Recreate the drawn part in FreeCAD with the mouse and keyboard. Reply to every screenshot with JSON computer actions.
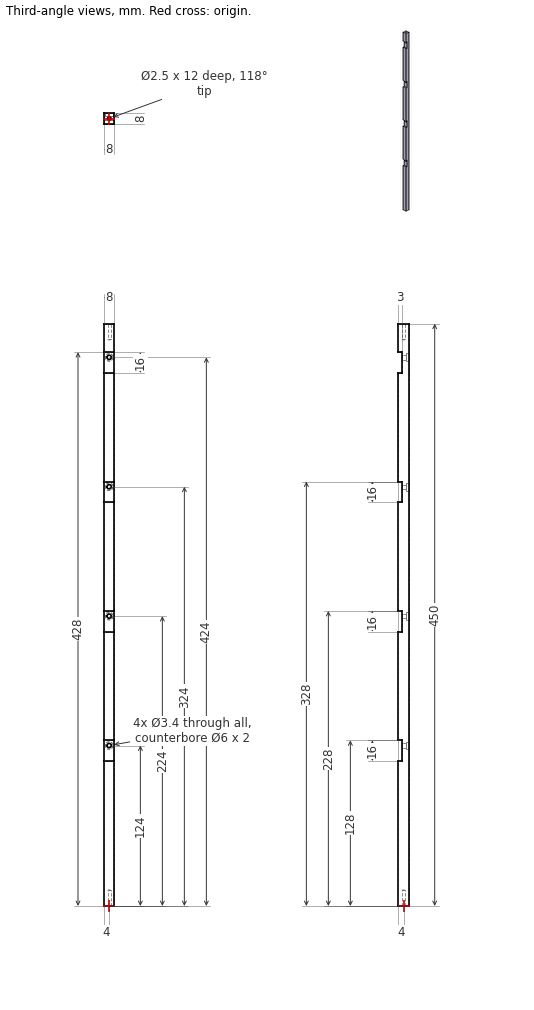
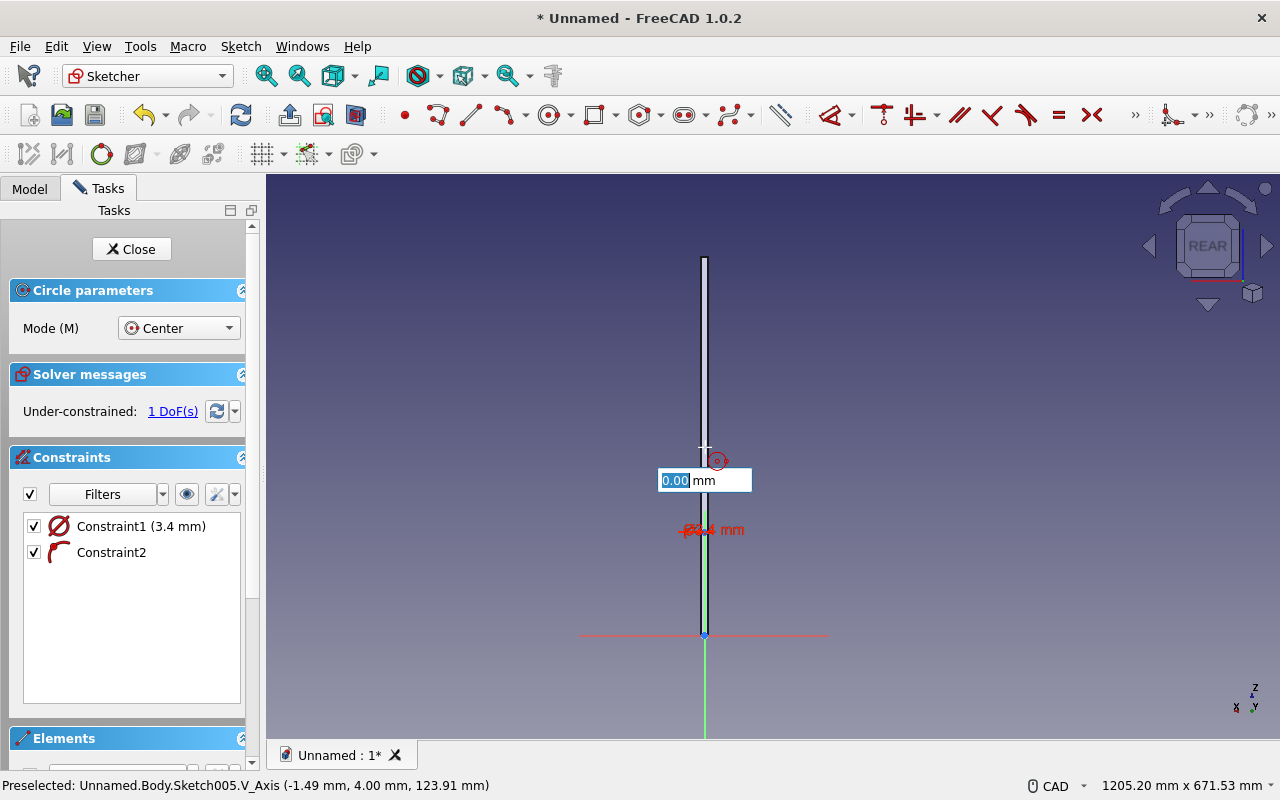
{"action": "scroll", "coordinate": [706, 447], "scroll_direction": "up", "scroll_amount": 13}
{"action": "mouse_move", "coordinate": [699, 436]}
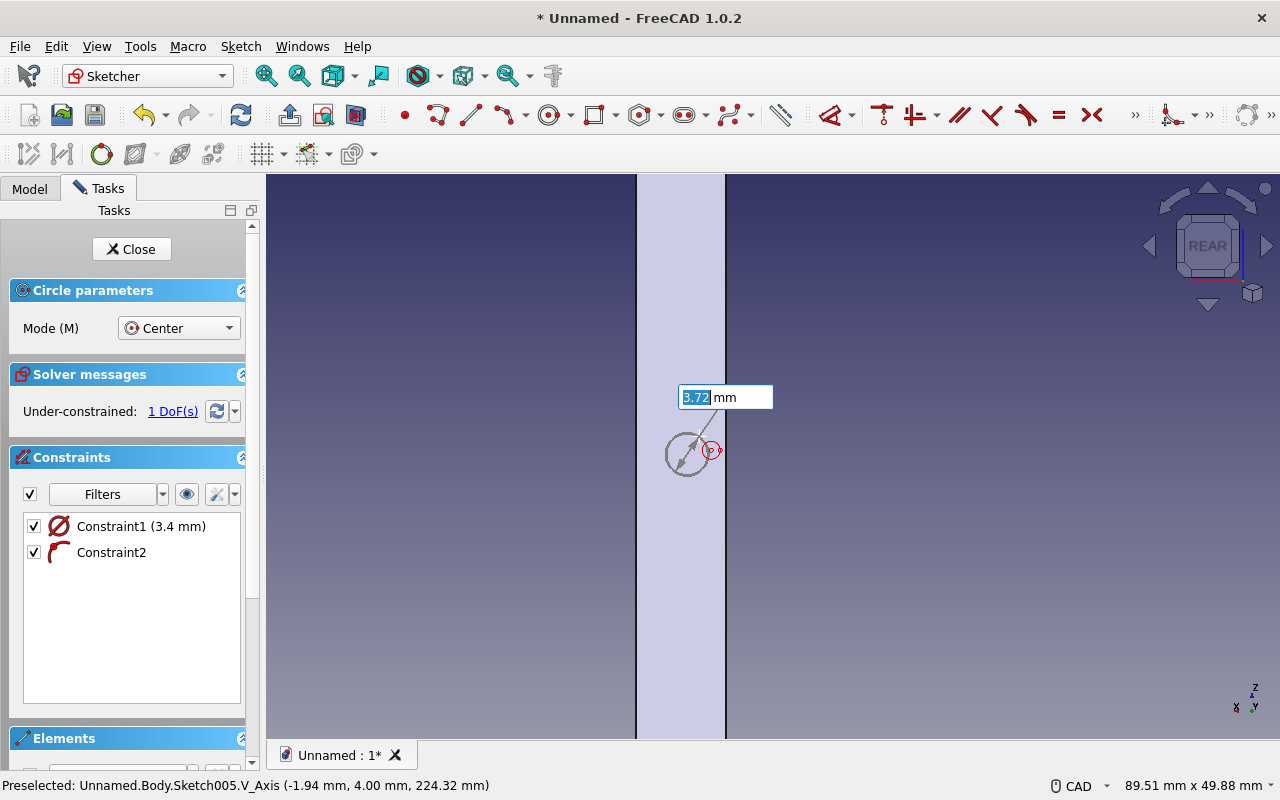
{"action": "type", "text": "3.4"}
{"action": "key", "text": "Return"}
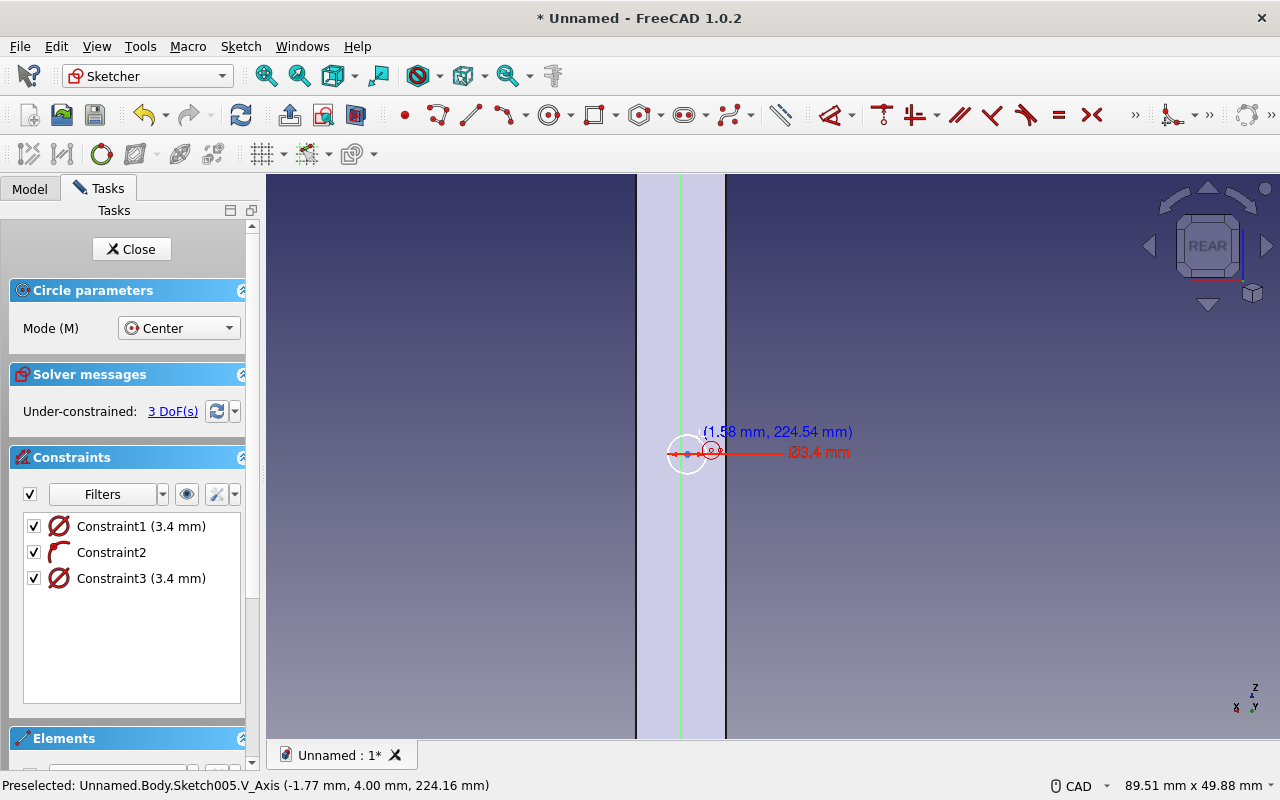
{"action": "scroll", "coordinate": [706, 447], "scroll_direction": "down", "scroll_amount": 13}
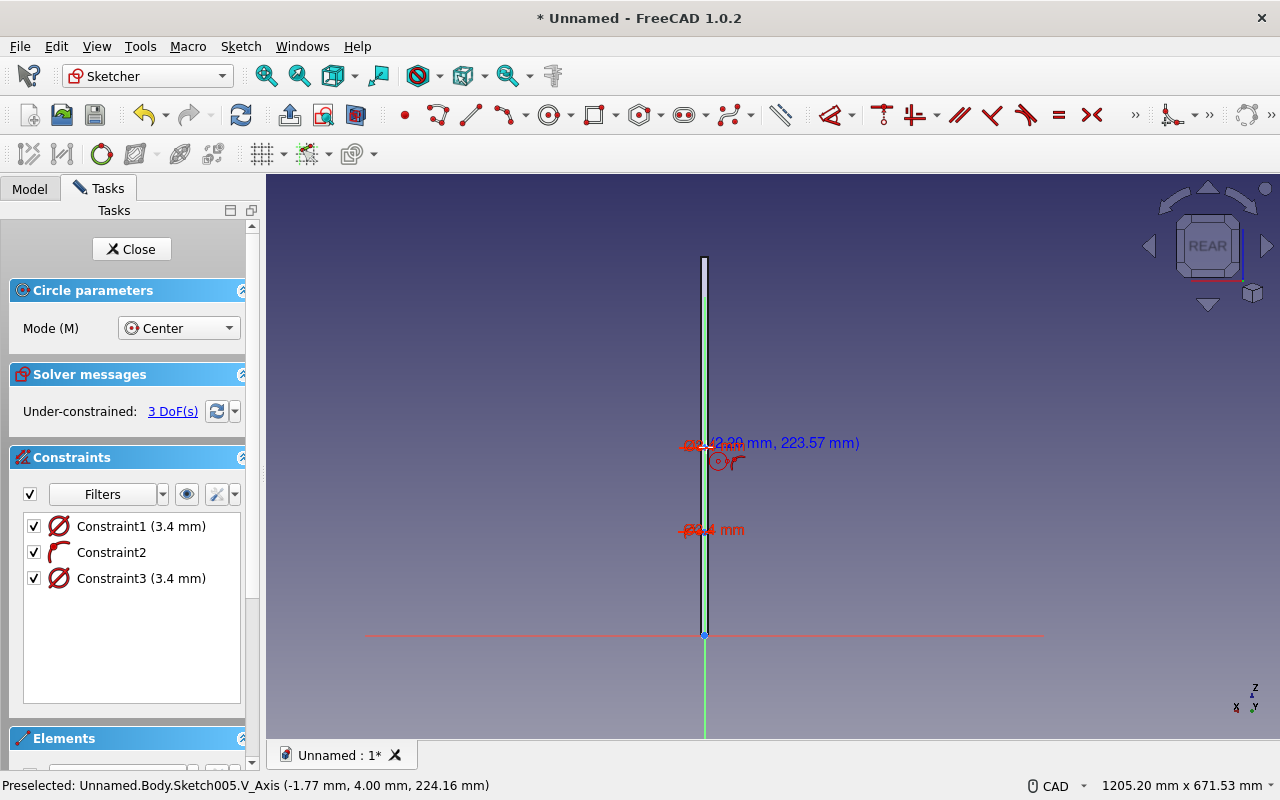
{"action": "scroll", "coordinate": [705, 363], "scroll_direction": "up", "scroll_amount": 14}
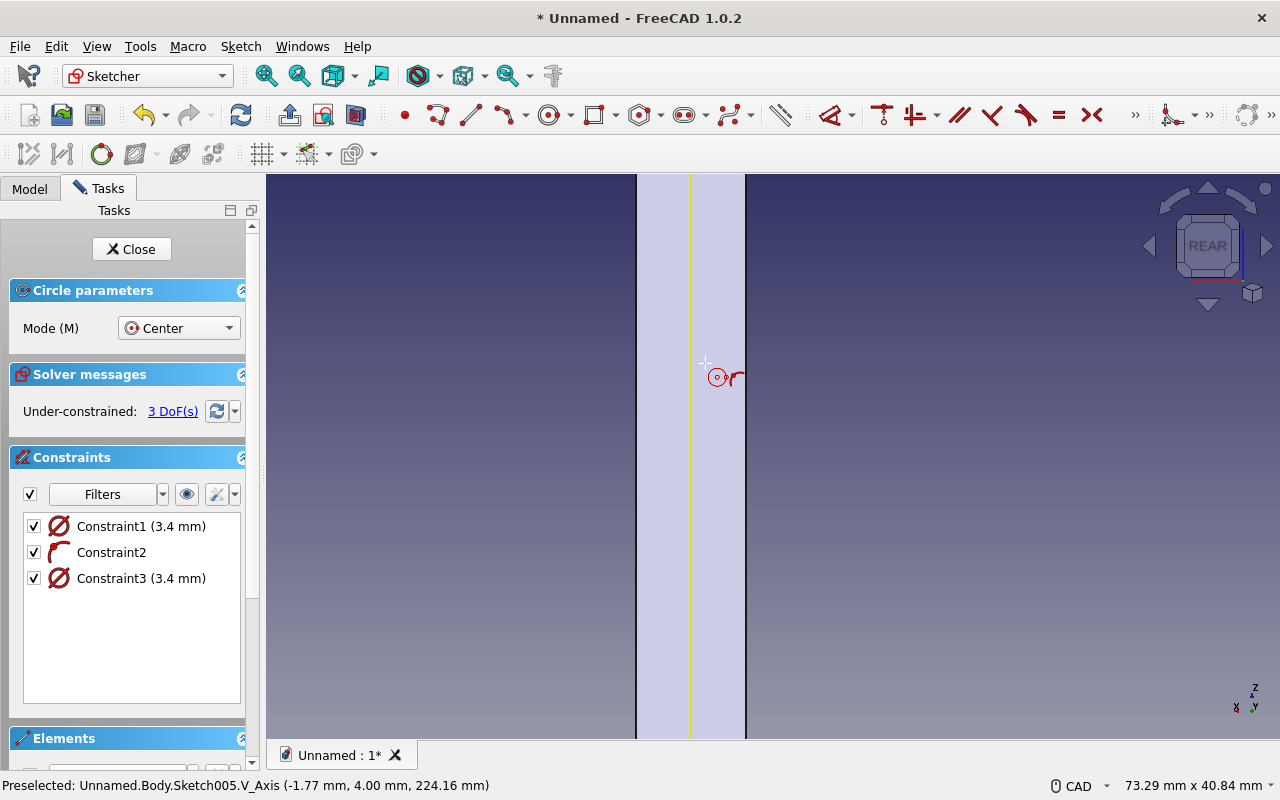
{"action": "scroll", "coordinate": [705, 363], "scroll_direction": "down", "scroll_amount": 14}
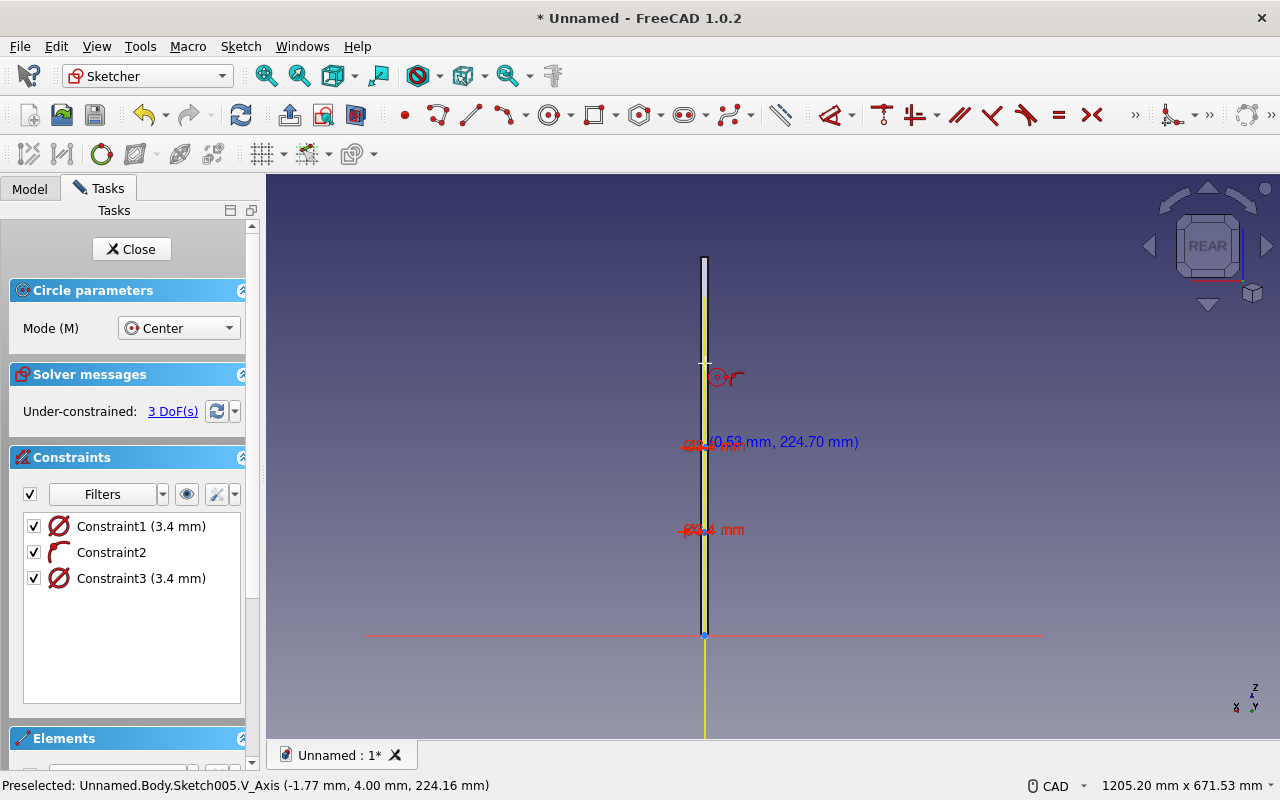
{"action": "left_click", "coordinate": [705, 363]}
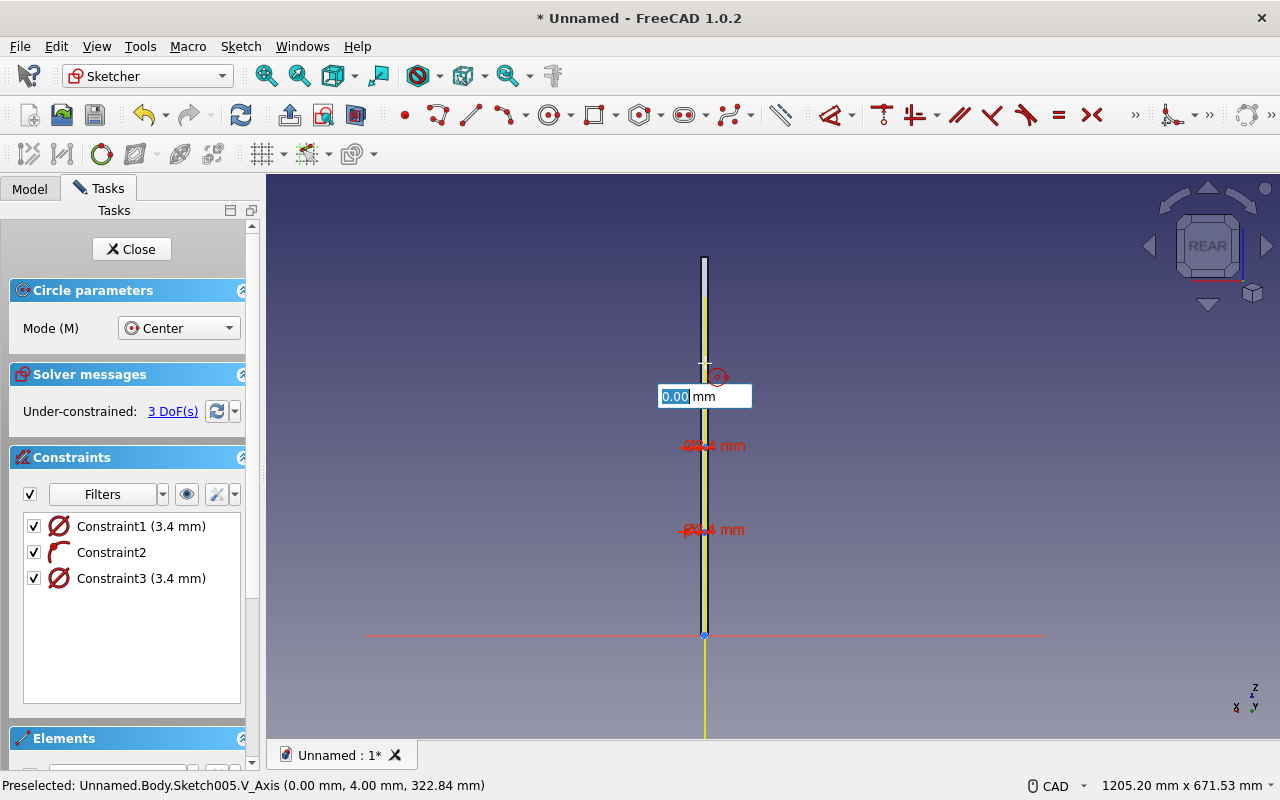
{"action": "scroll", "coordinate": [706, 363], "scroll_direction": "up", "scroll_amount": 13}
{"action": "mouse_move", "coordinate": [699, 353]}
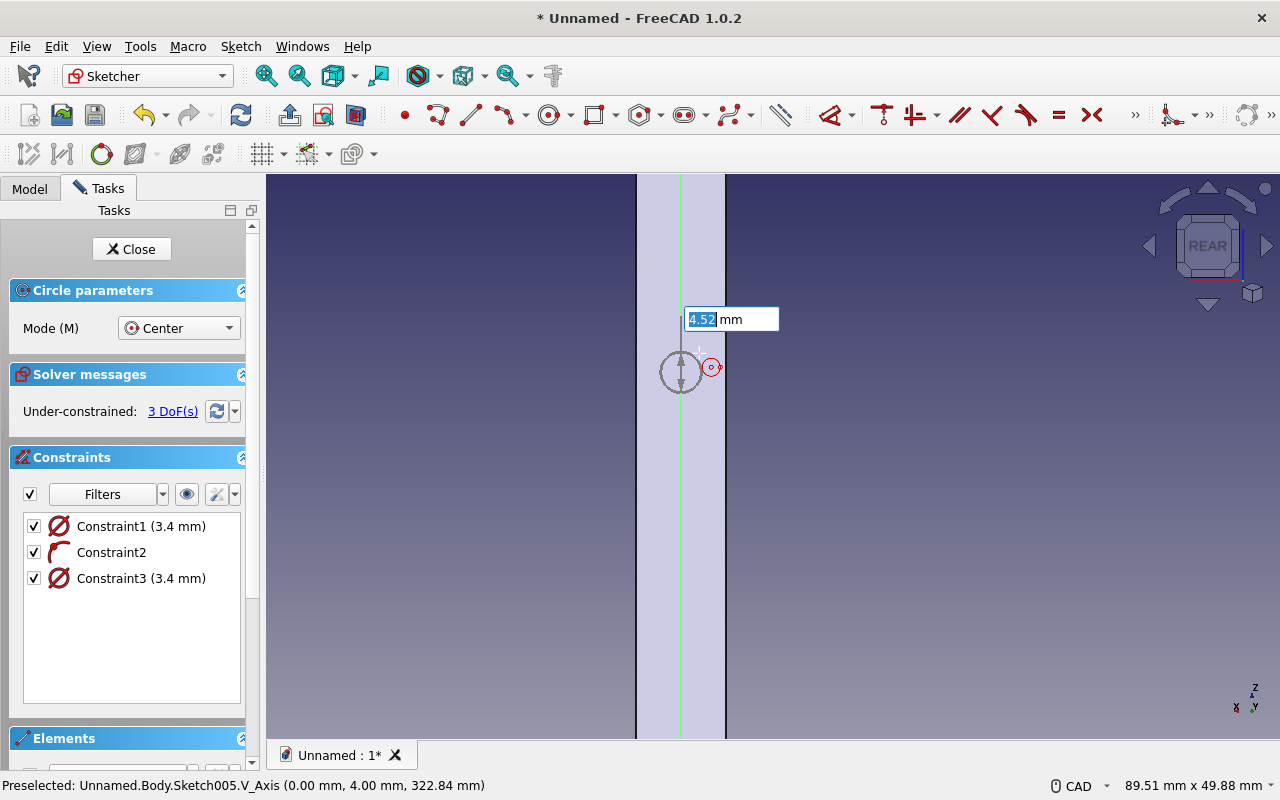
{"action": "type", "text": "3.4"}
{"action": "key", "text": "Return"}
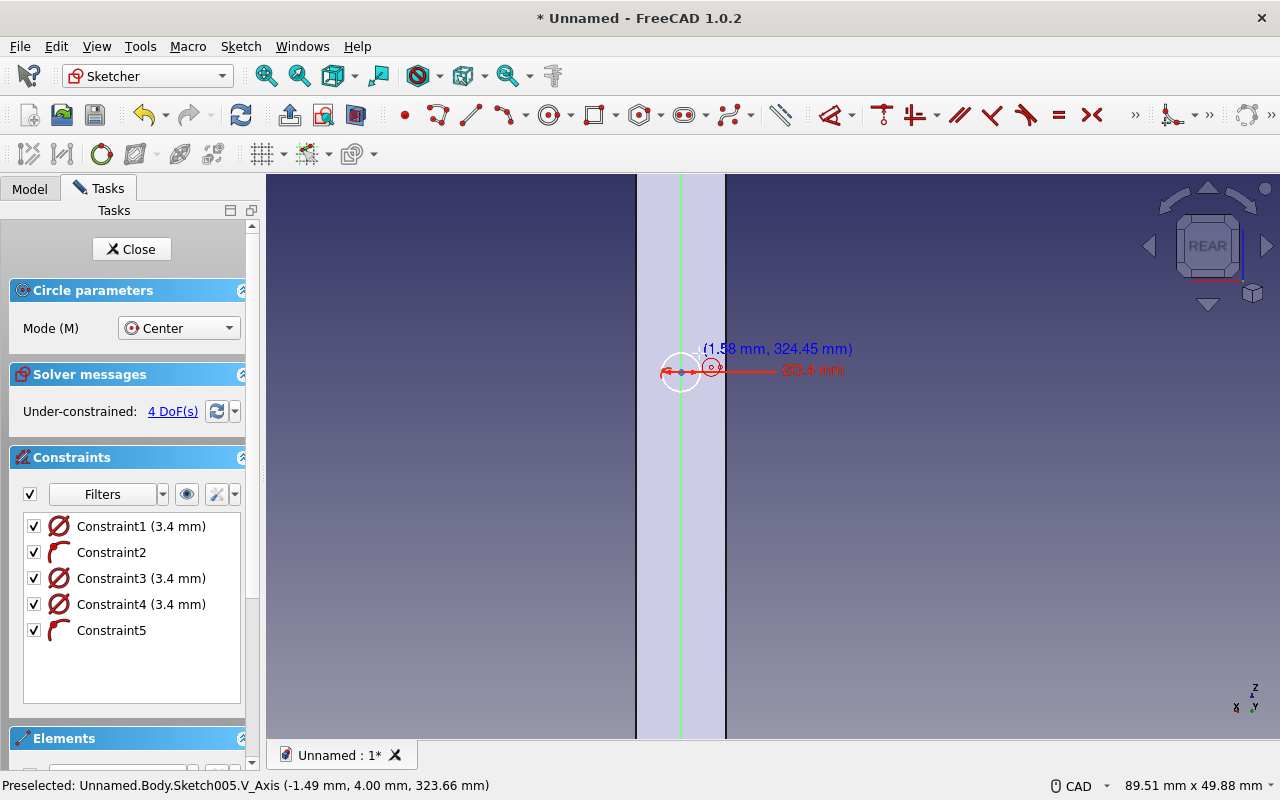
{"action": "scroll", "coordinate": [706, 363], "scroll_direction": "down", "scroll_amount": 13}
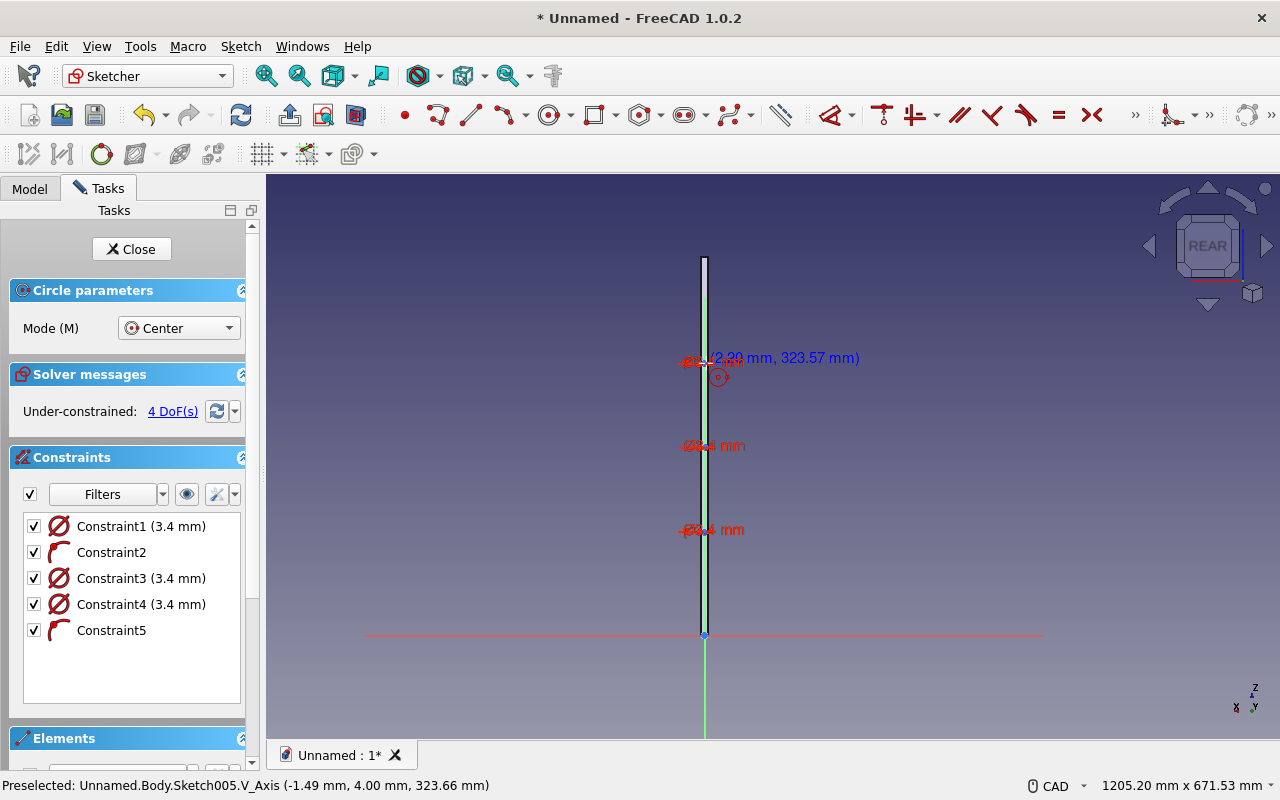
{"action": "scroll", "coordinate": [705, 279], "scroll_direction": "up", "scroll_amount": 14}